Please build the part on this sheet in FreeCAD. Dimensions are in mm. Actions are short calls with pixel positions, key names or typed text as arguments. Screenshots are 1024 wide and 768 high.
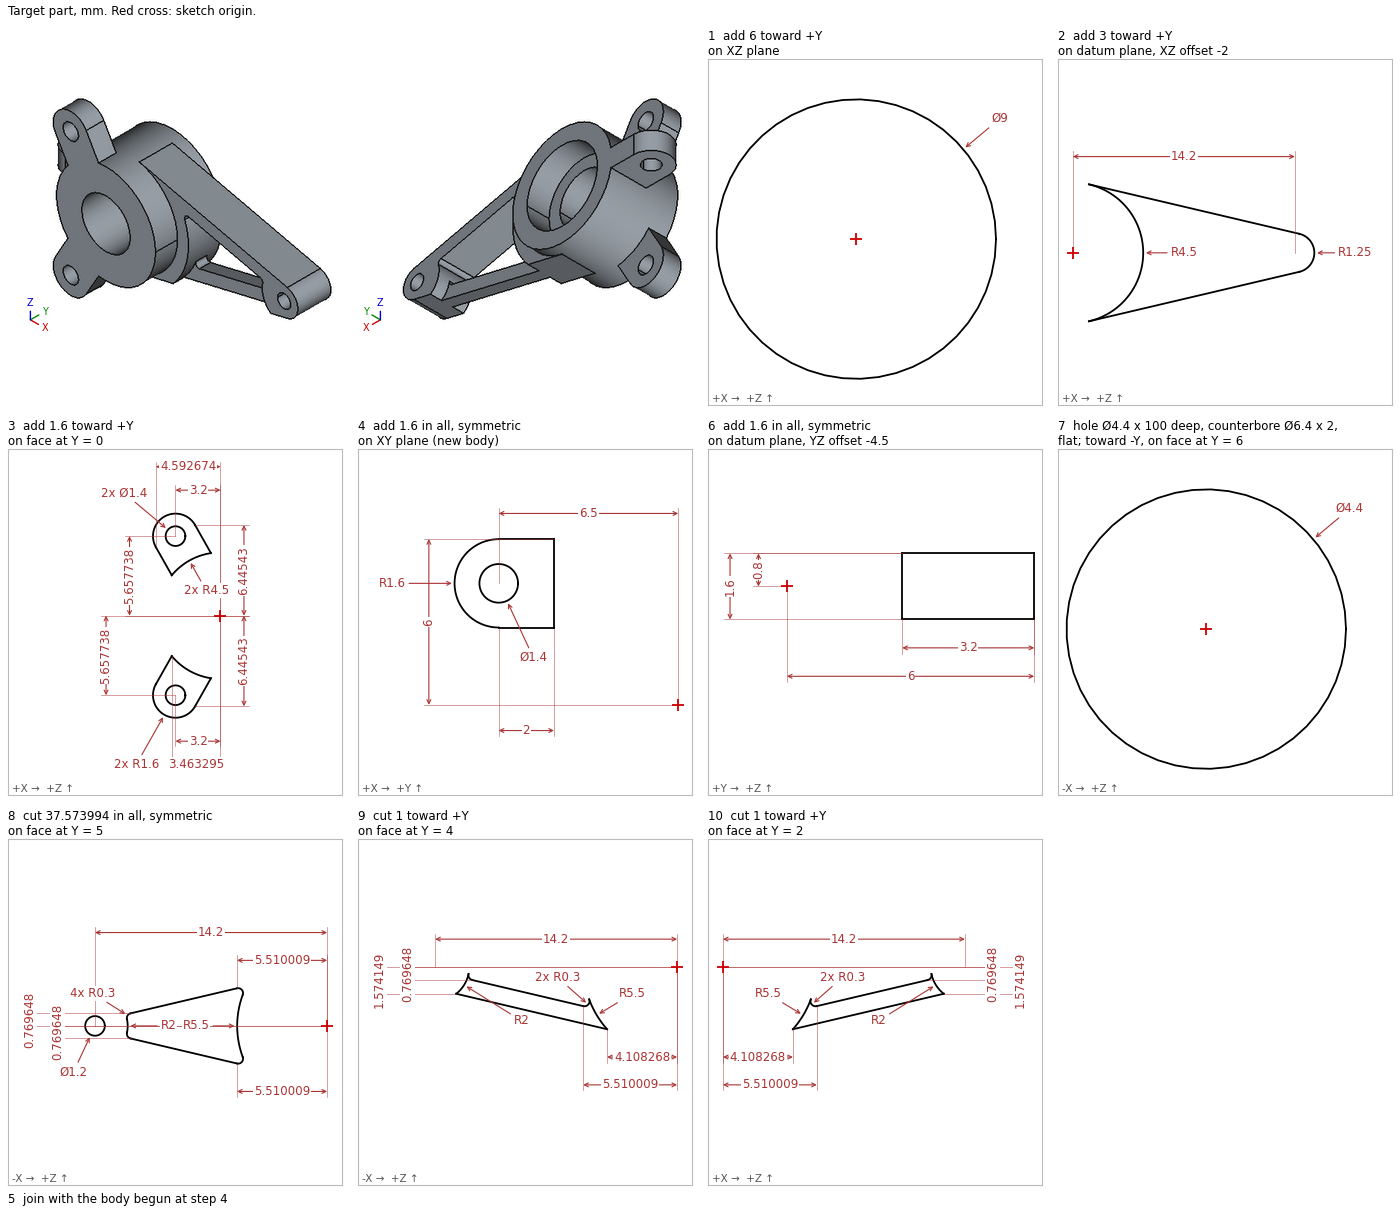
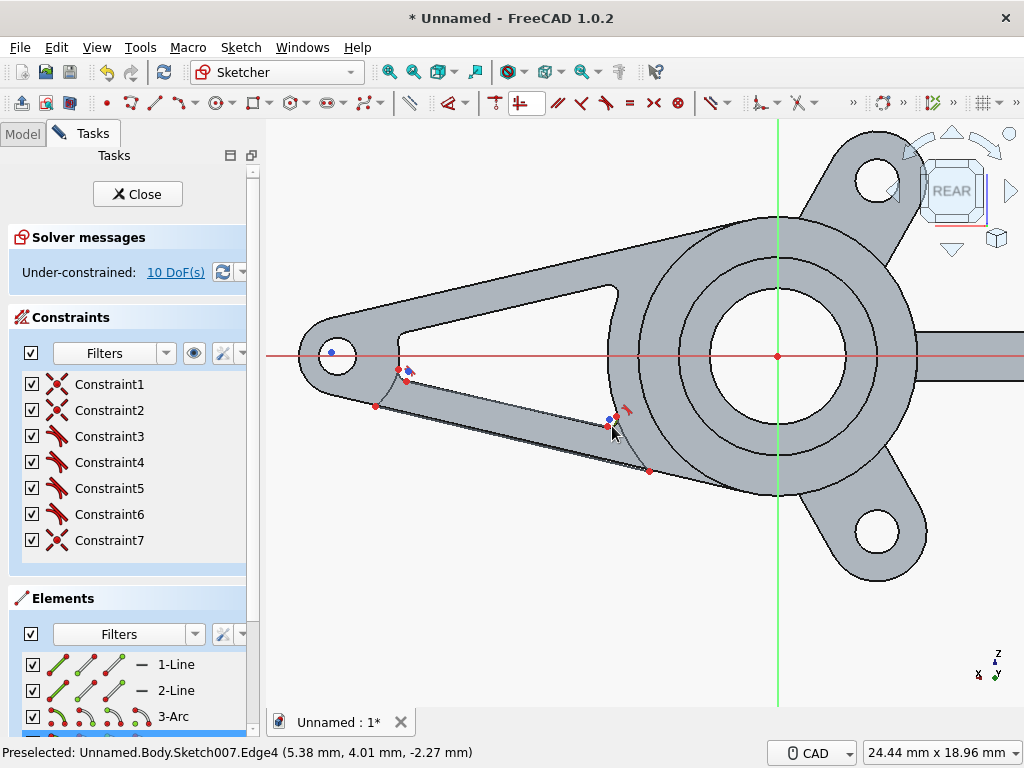
scroll(402, 379, up, 6)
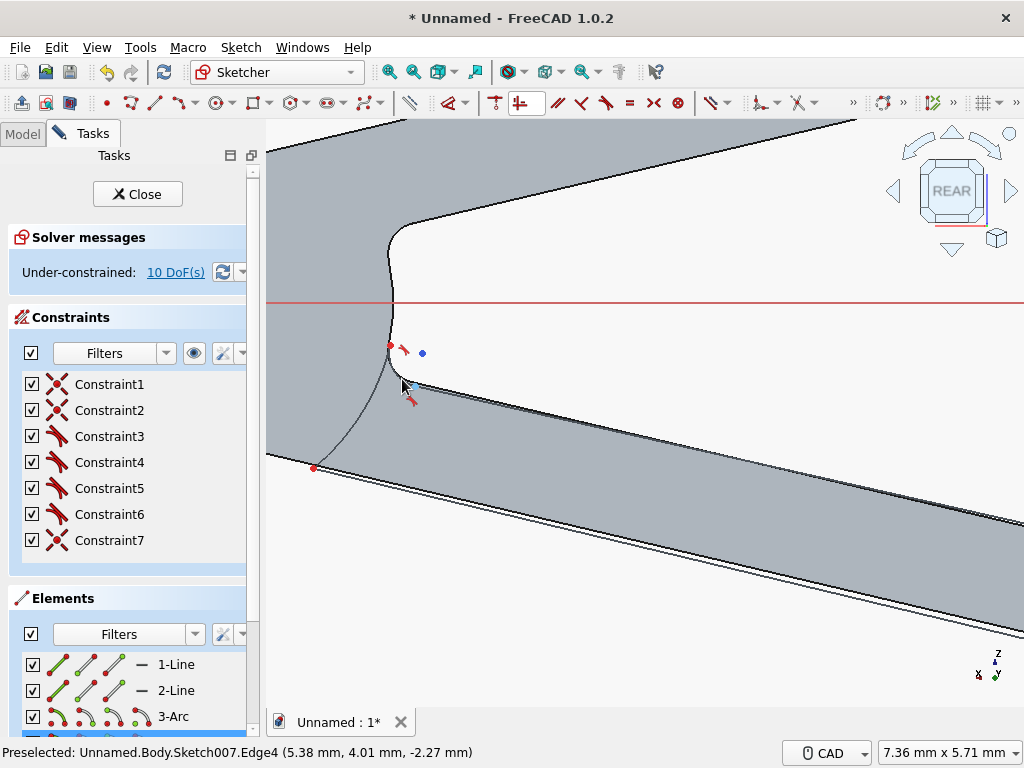
click(401, 379)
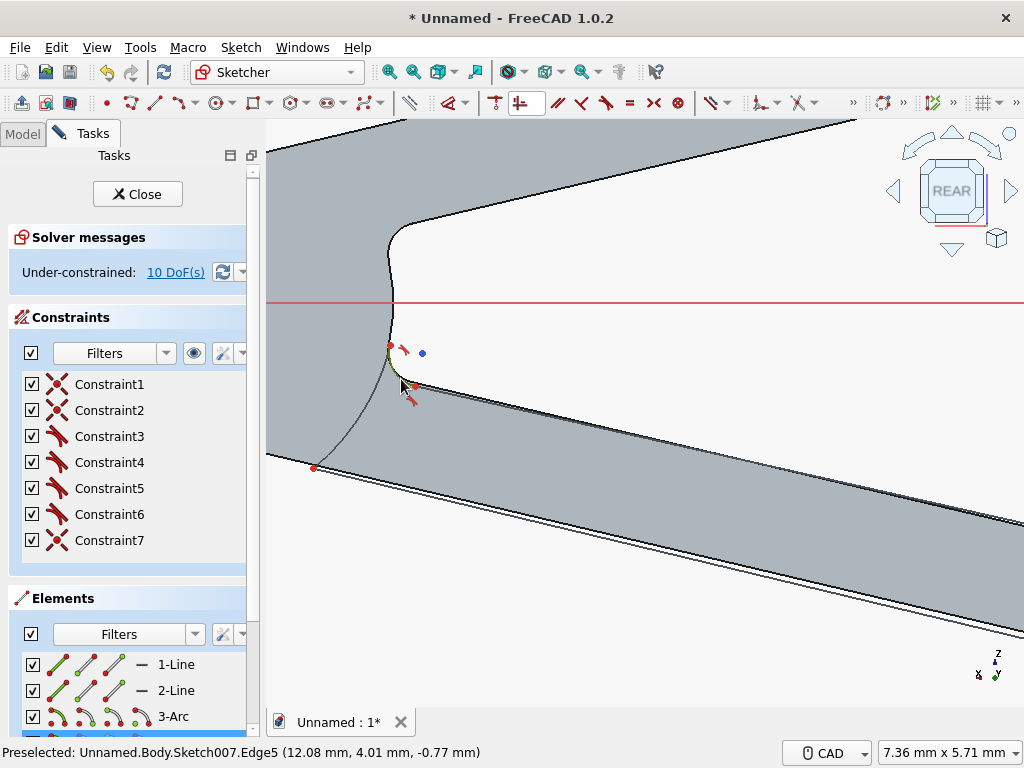
key(e)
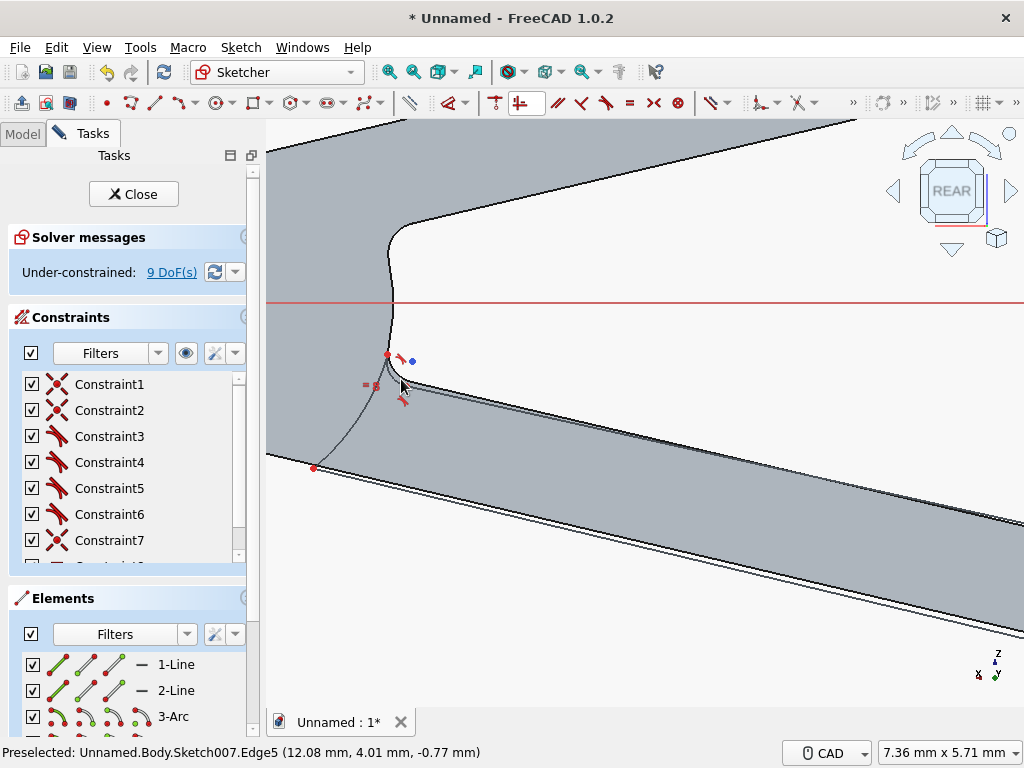
scroll(402, 379, down, 6)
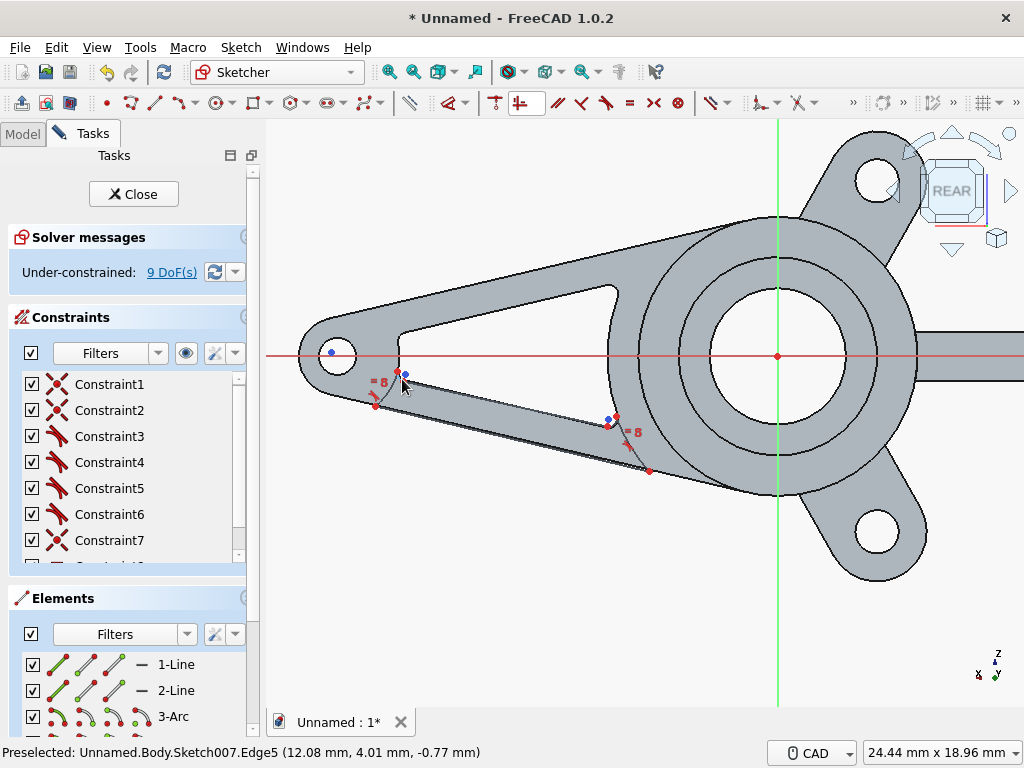
click(331, 353)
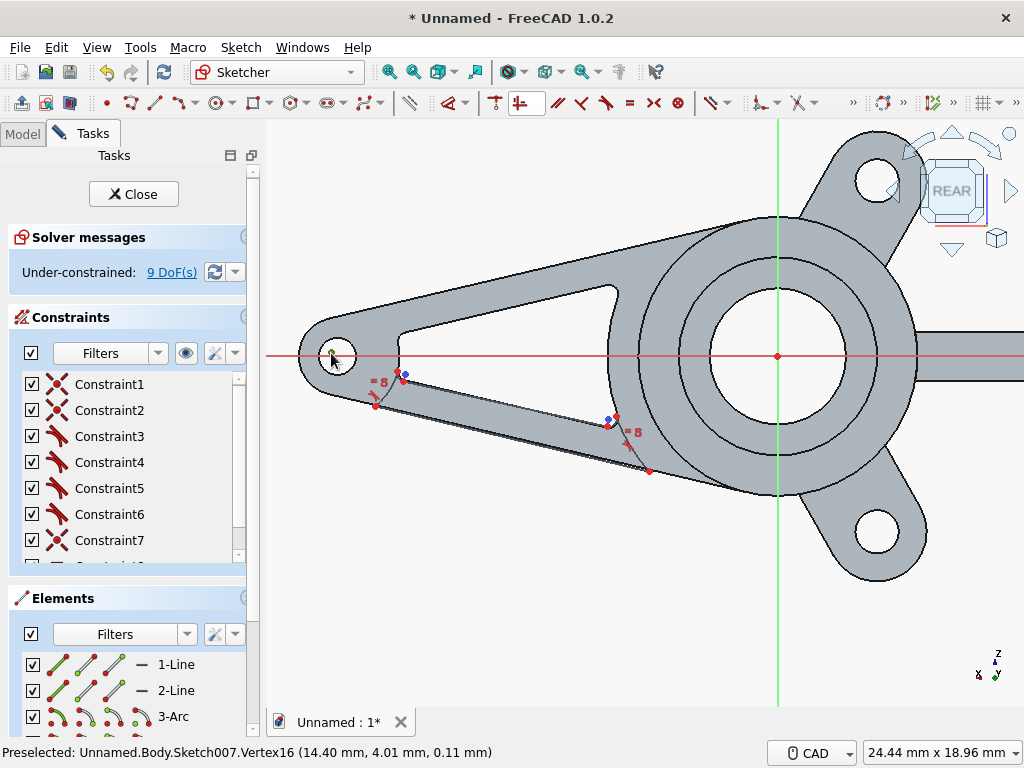
click(455, 356)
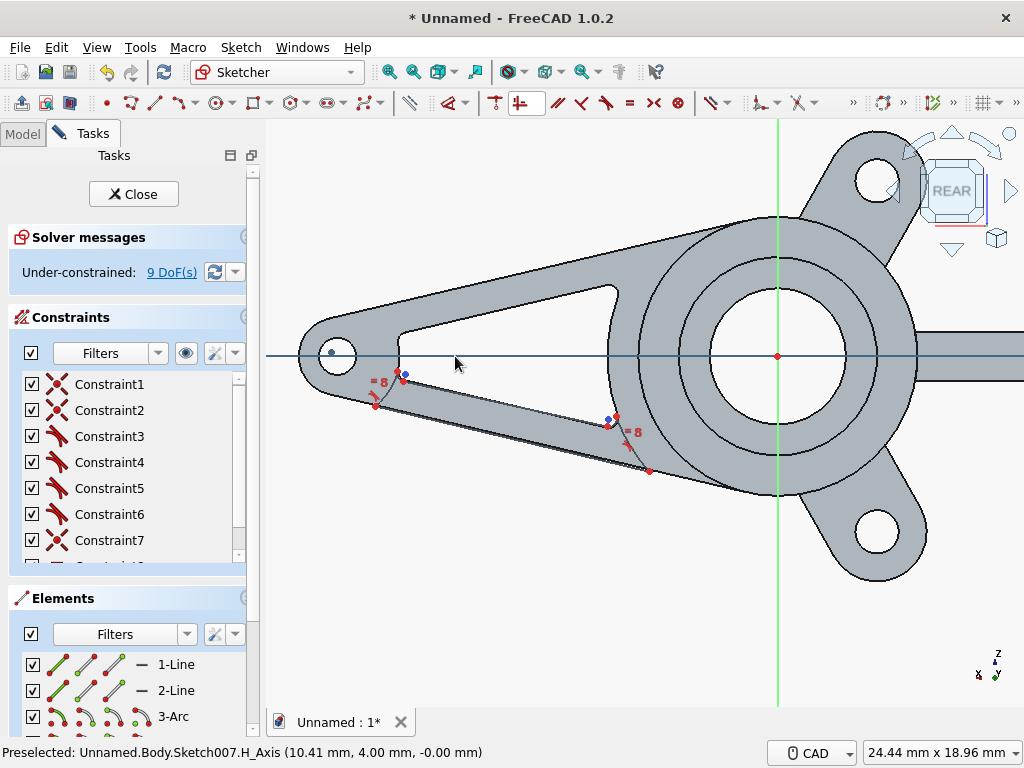
key(c)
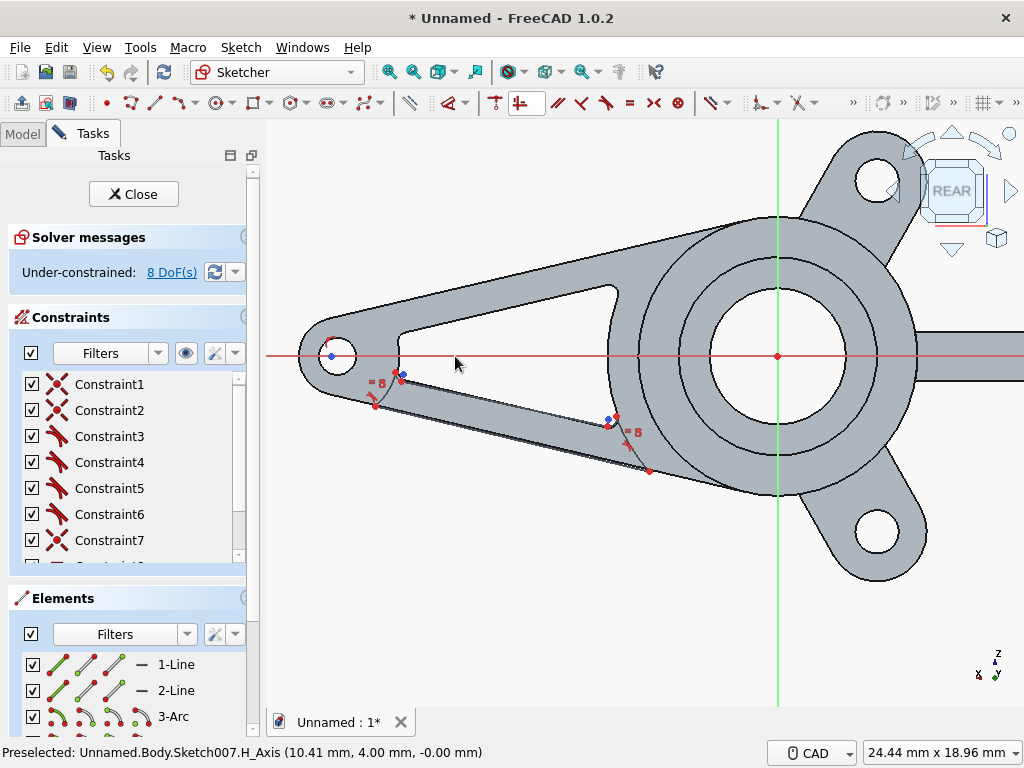
click(448, 104)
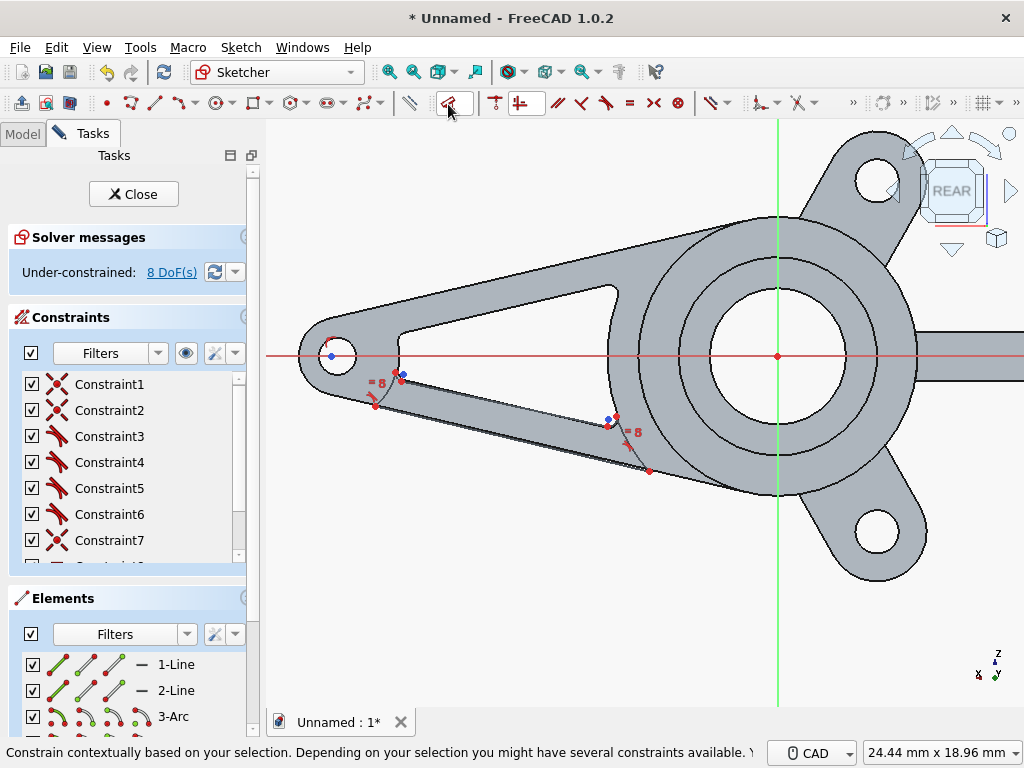
click(624, 434)
click(662, 525)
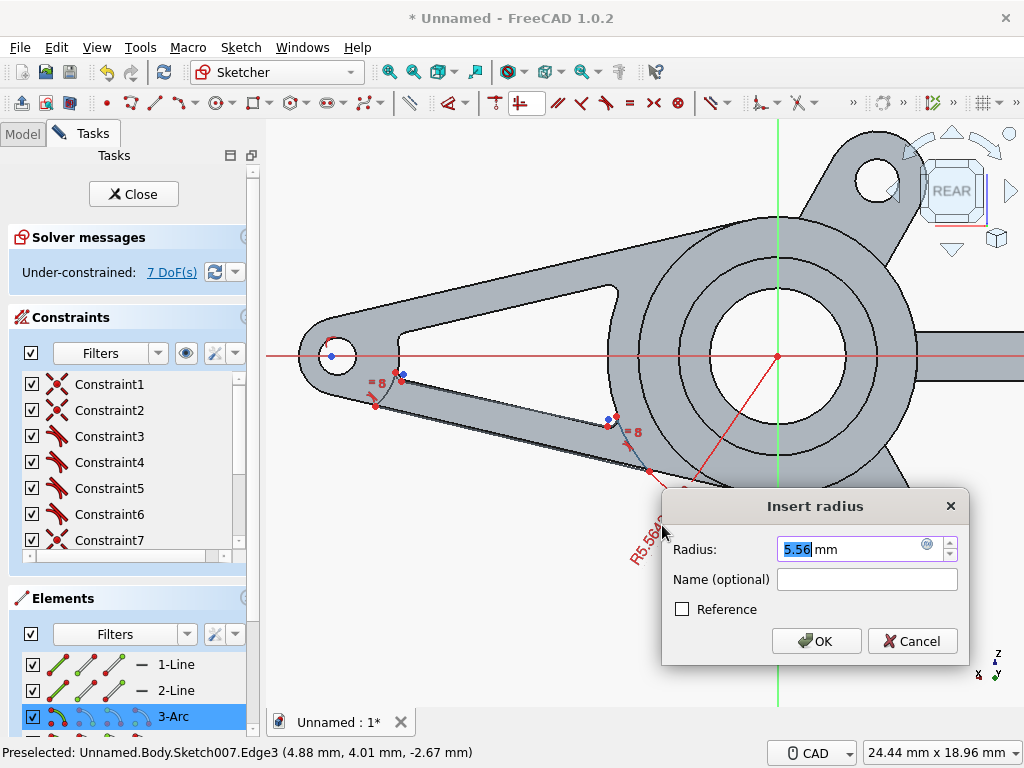
text(5.5)
key(Return)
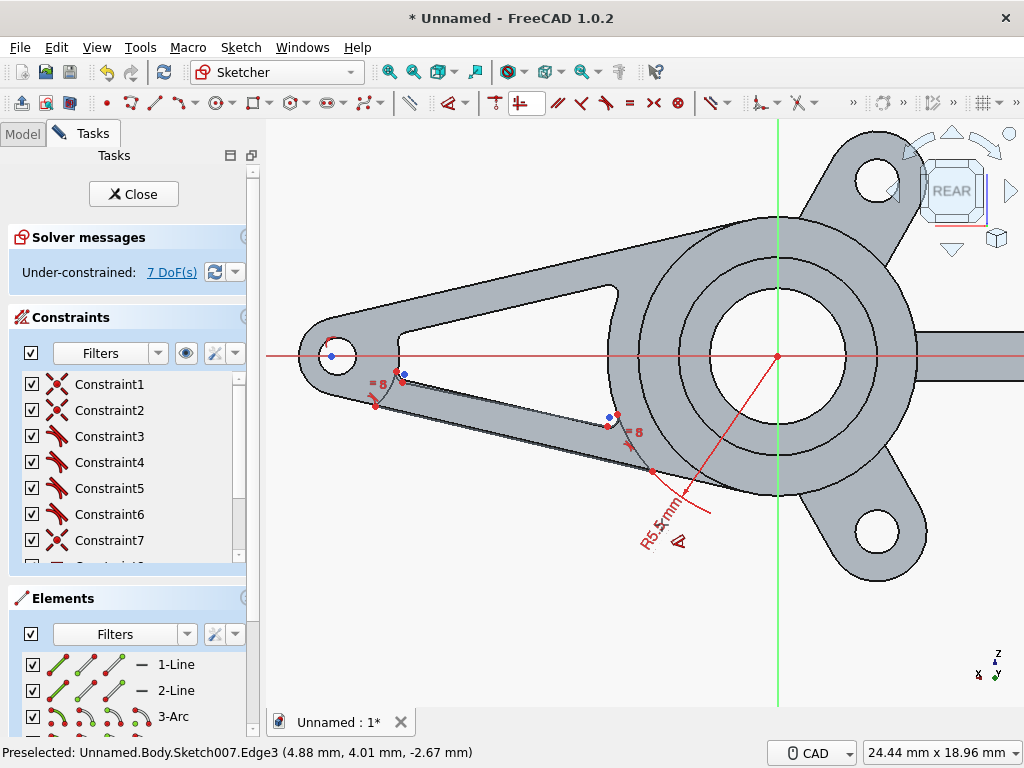
scroll(613, 426, up, 8)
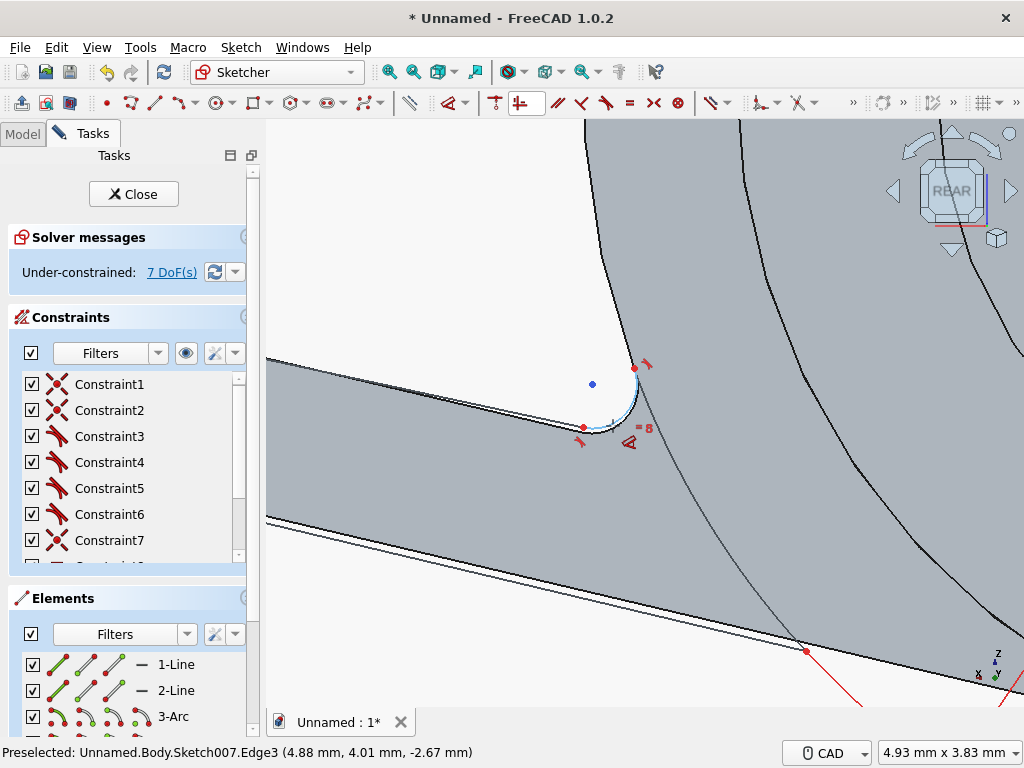
click(611, 425)
click(624, 454)